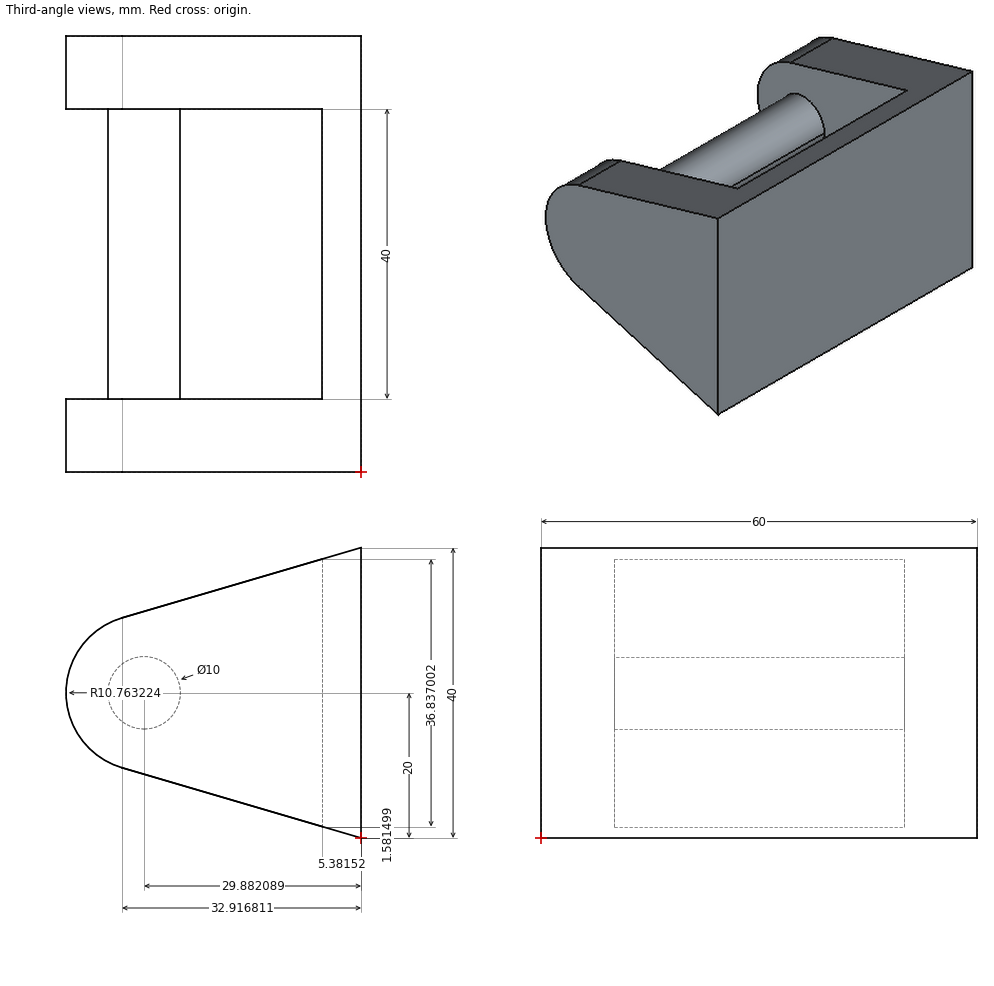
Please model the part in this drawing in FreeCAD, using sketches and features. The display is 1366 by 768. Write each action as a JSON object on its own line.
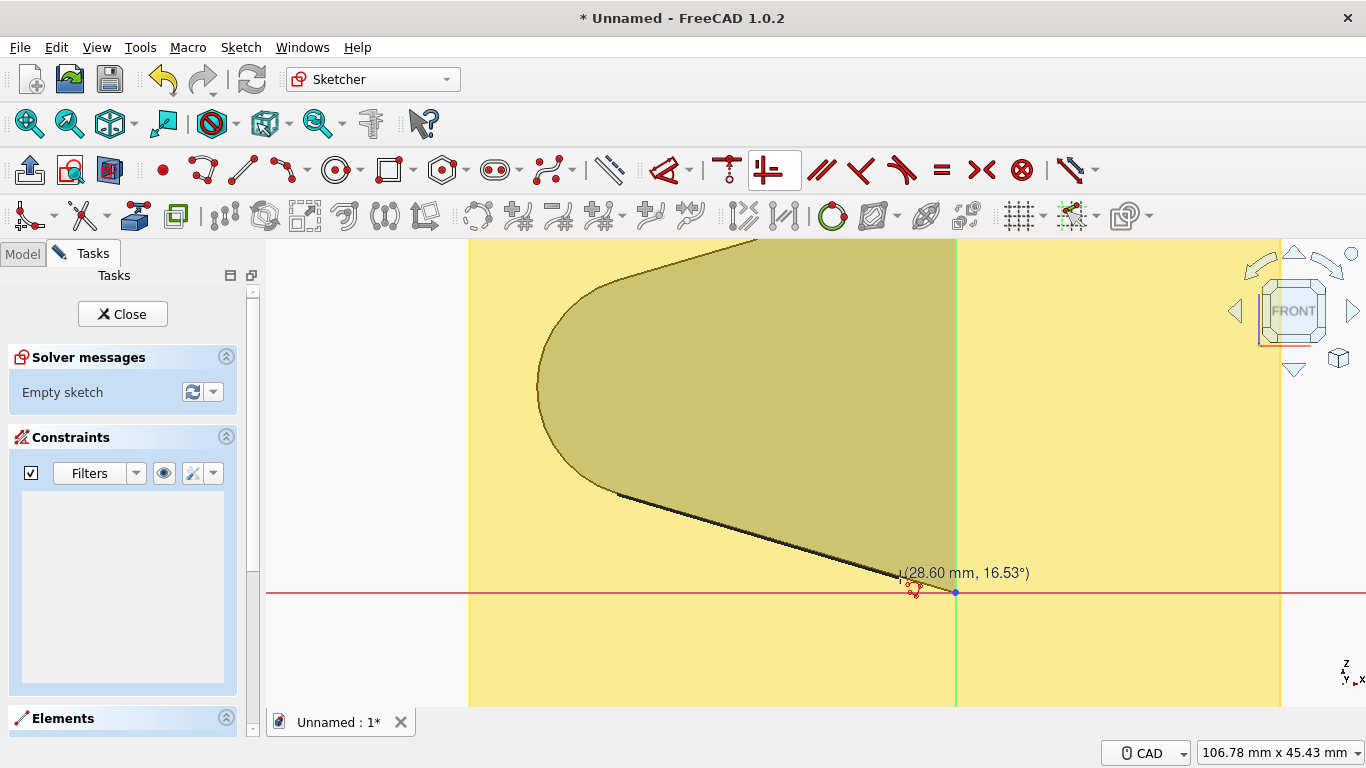
{"action": "left_click", "coordinate": [900, 577]}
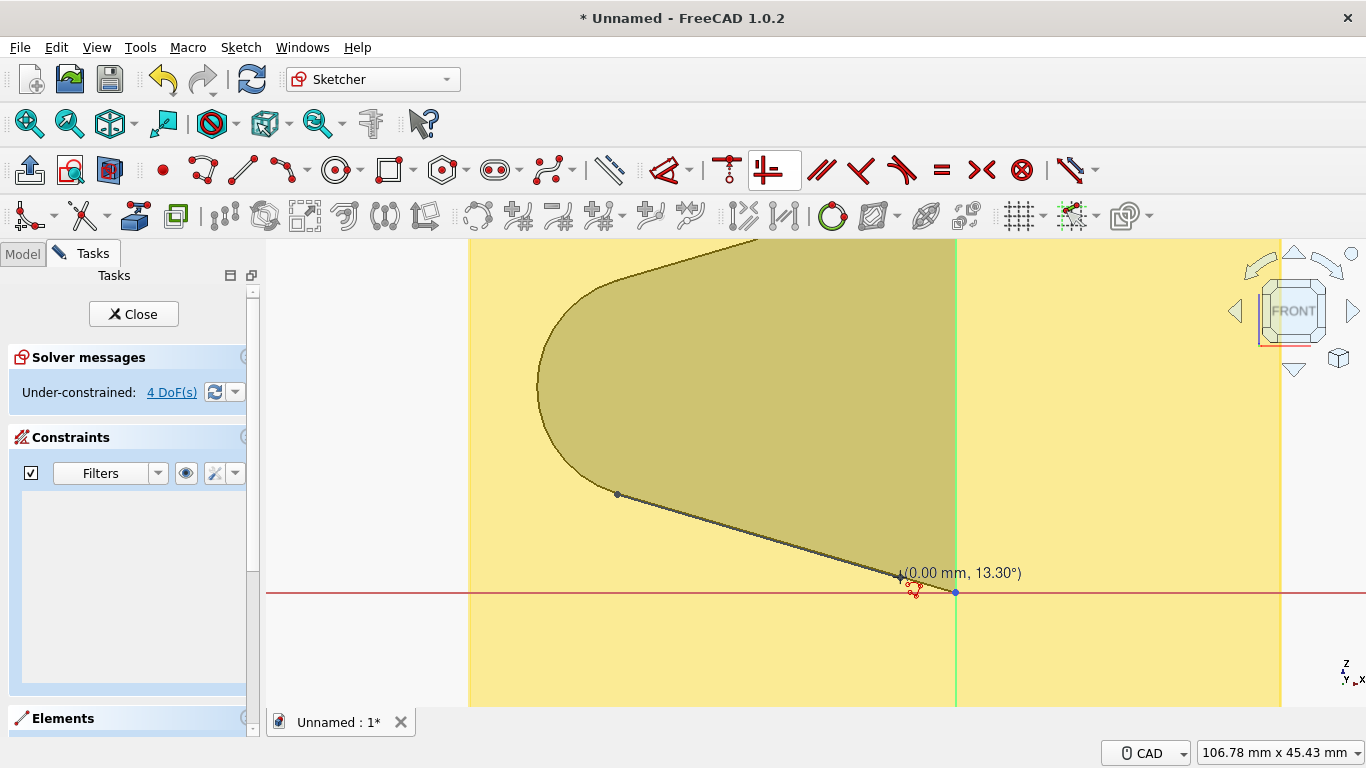
{"action": "scroll", "coordinate": [750, 631], "scroll_direction": "down", "scroll_amount": 2}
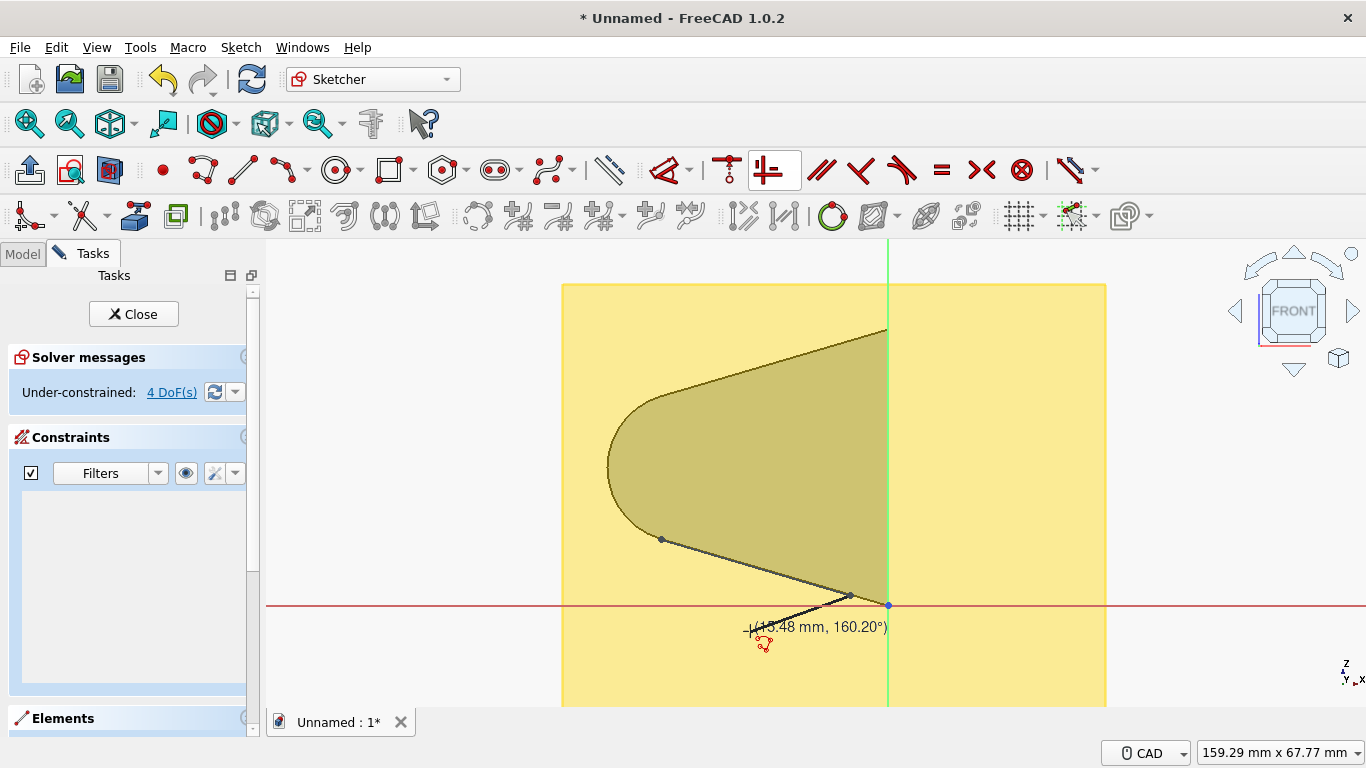
{"action": "left_click", "coordinate": [851, 340]}
{"action": "left_click", "coordinate": [661, 396]}
{"action": "right_click", "coordinate": [661, 396]}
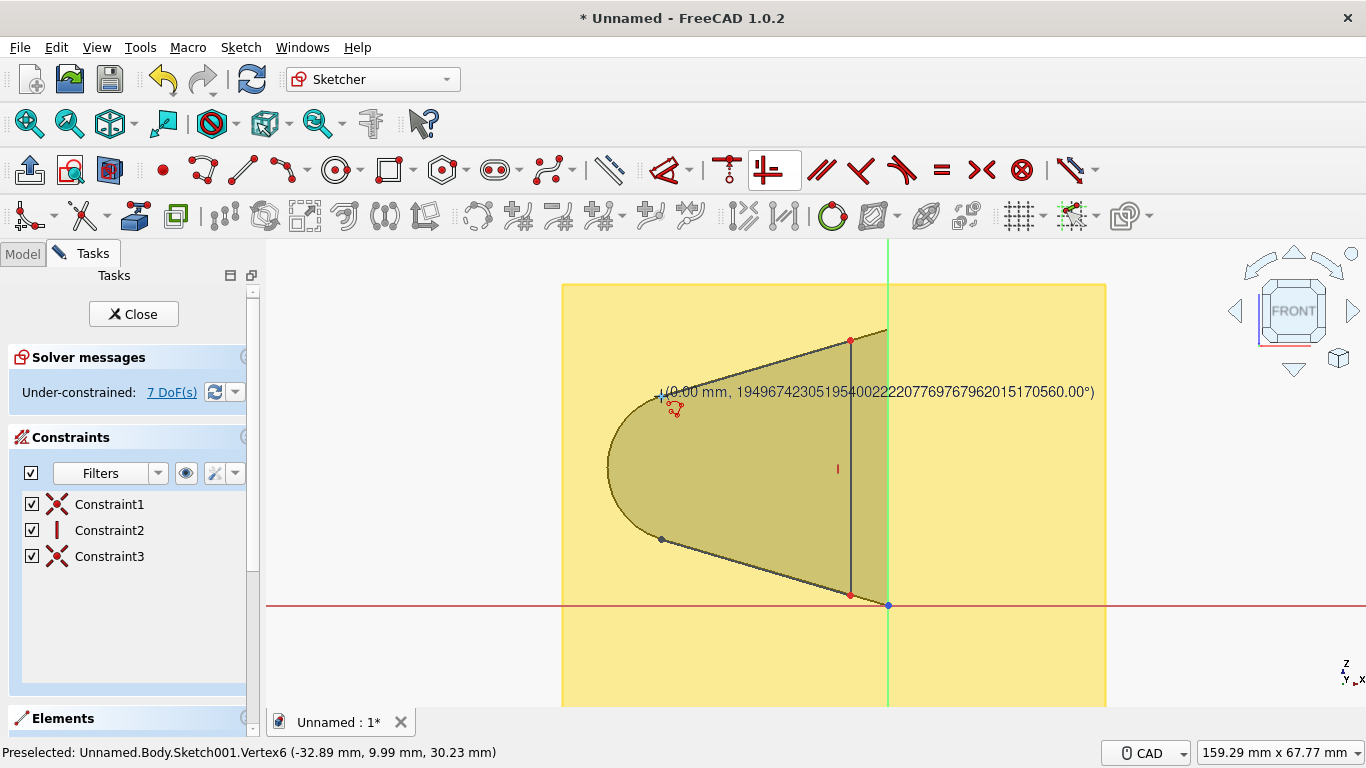
{"action": "left_click", "coordinate": [284, 170]}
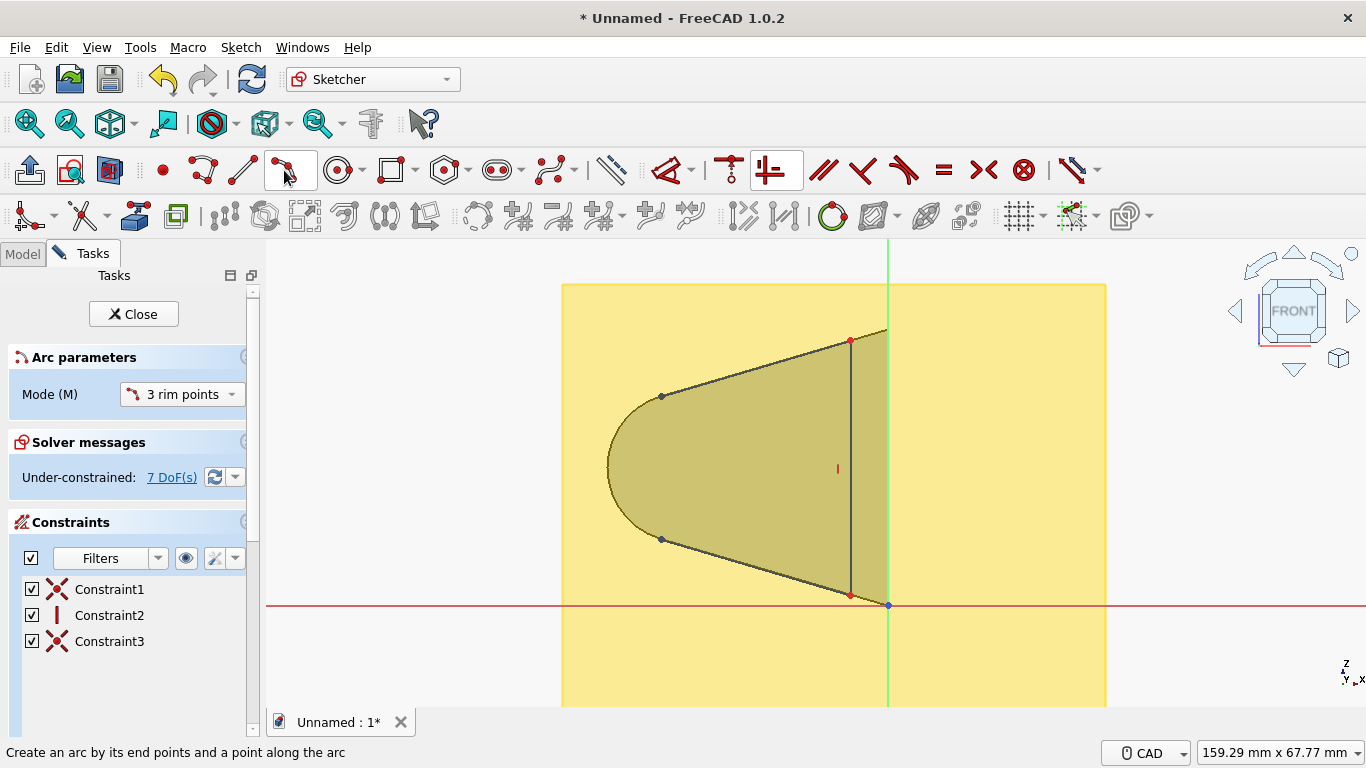
{"action": "left_click", "coordinate": [661, 397]}
{"action": "left_click", "coordinate": [661, 540]}
{"action": "left_click", "coordinate": [607, 468]}
{"action": "key", "text": "Escape"}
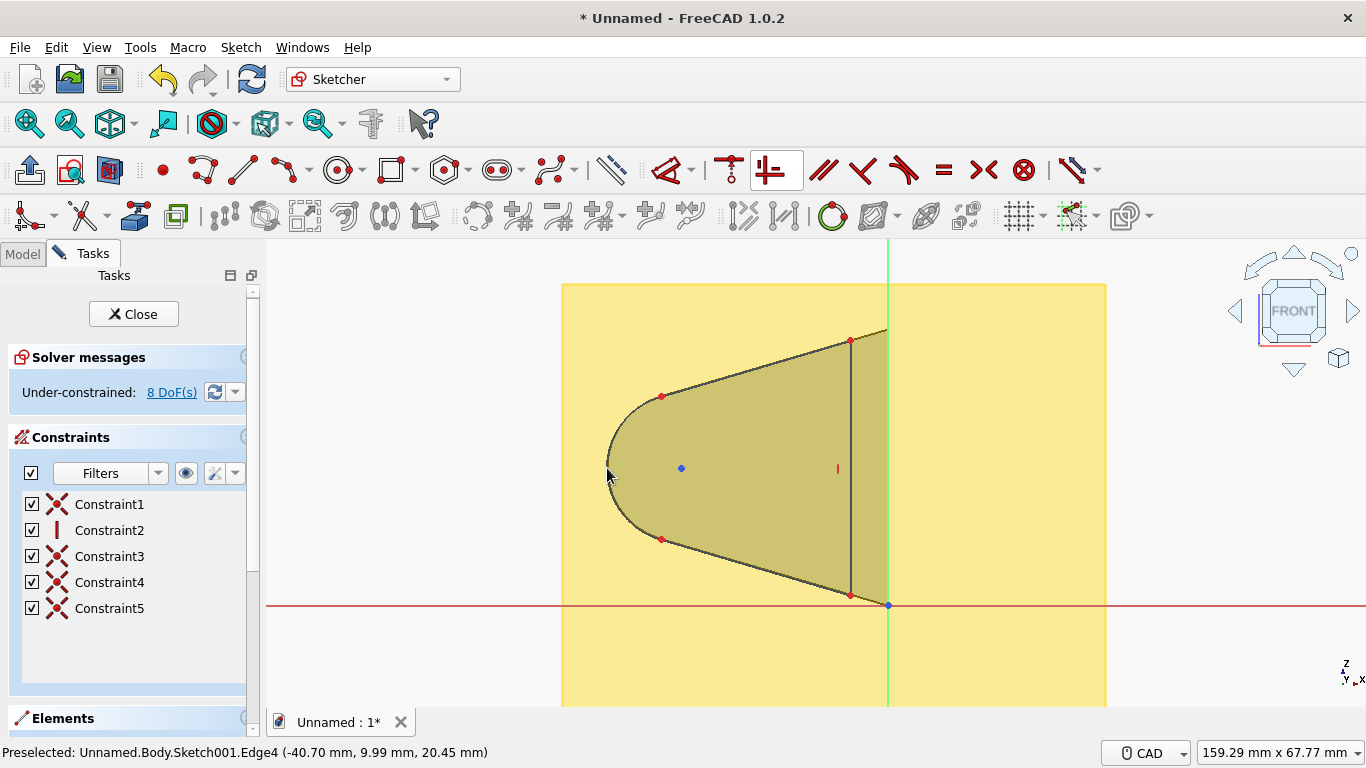
{"action": "left_click", "coordinate": [718, 557]}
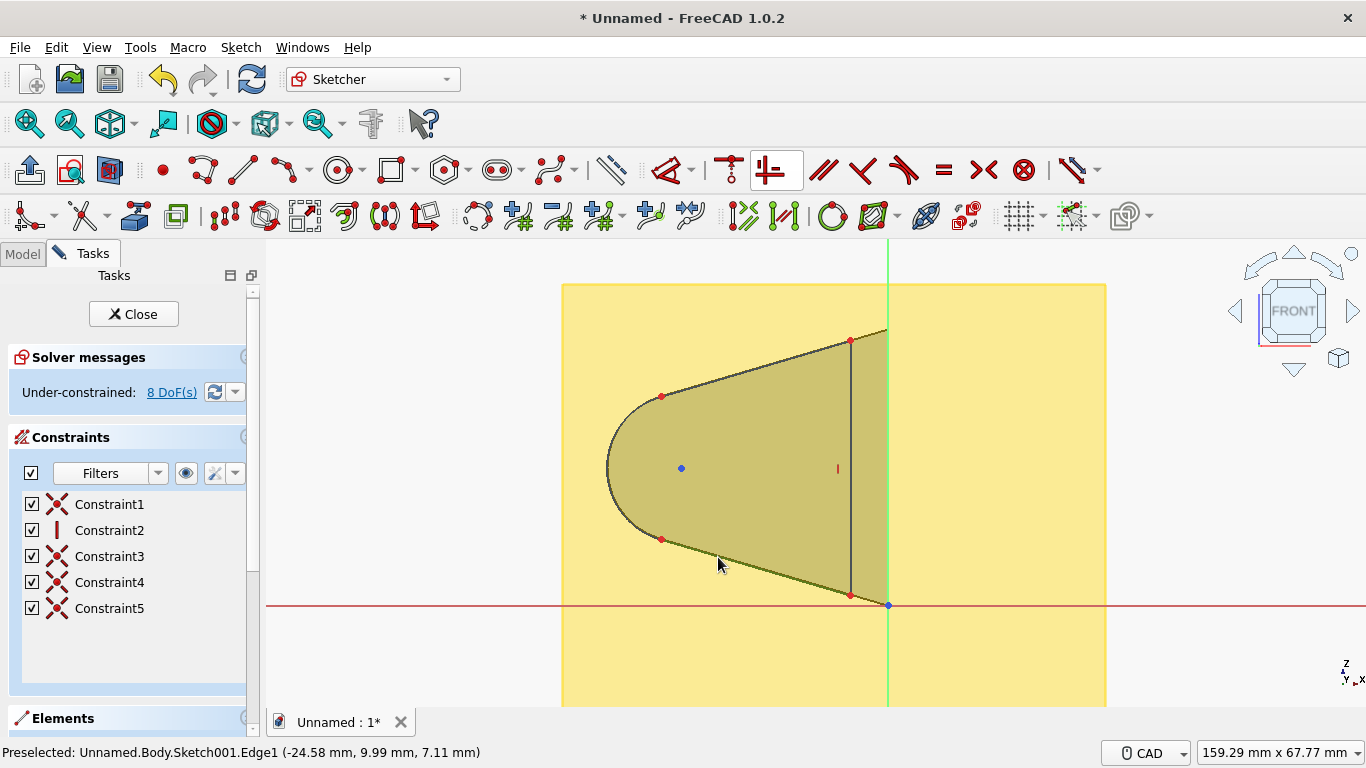
{"action": "left_click", "coordinate": [617, 432]}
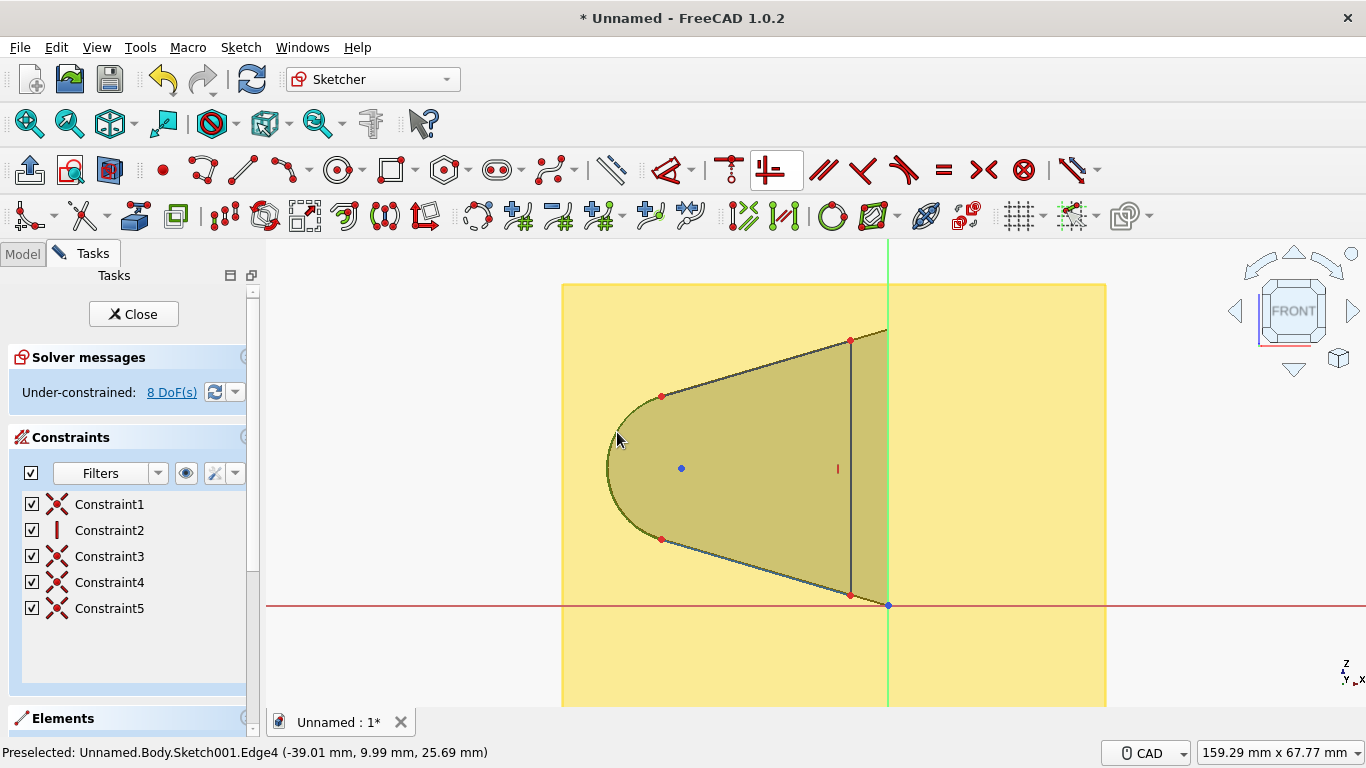
{"action": "left_click", "coordinate": [904, 170]}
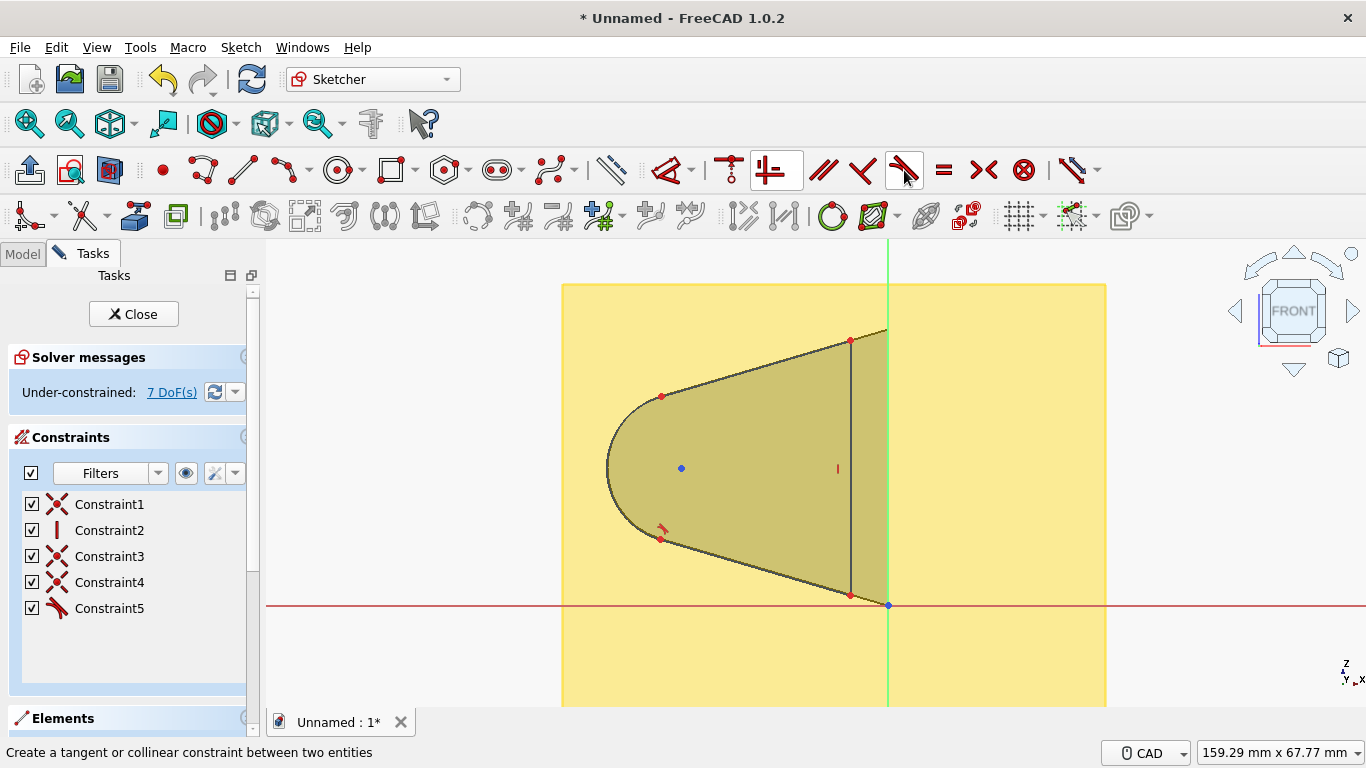
{"action": "left_click", "coordinate": [794, 358]}